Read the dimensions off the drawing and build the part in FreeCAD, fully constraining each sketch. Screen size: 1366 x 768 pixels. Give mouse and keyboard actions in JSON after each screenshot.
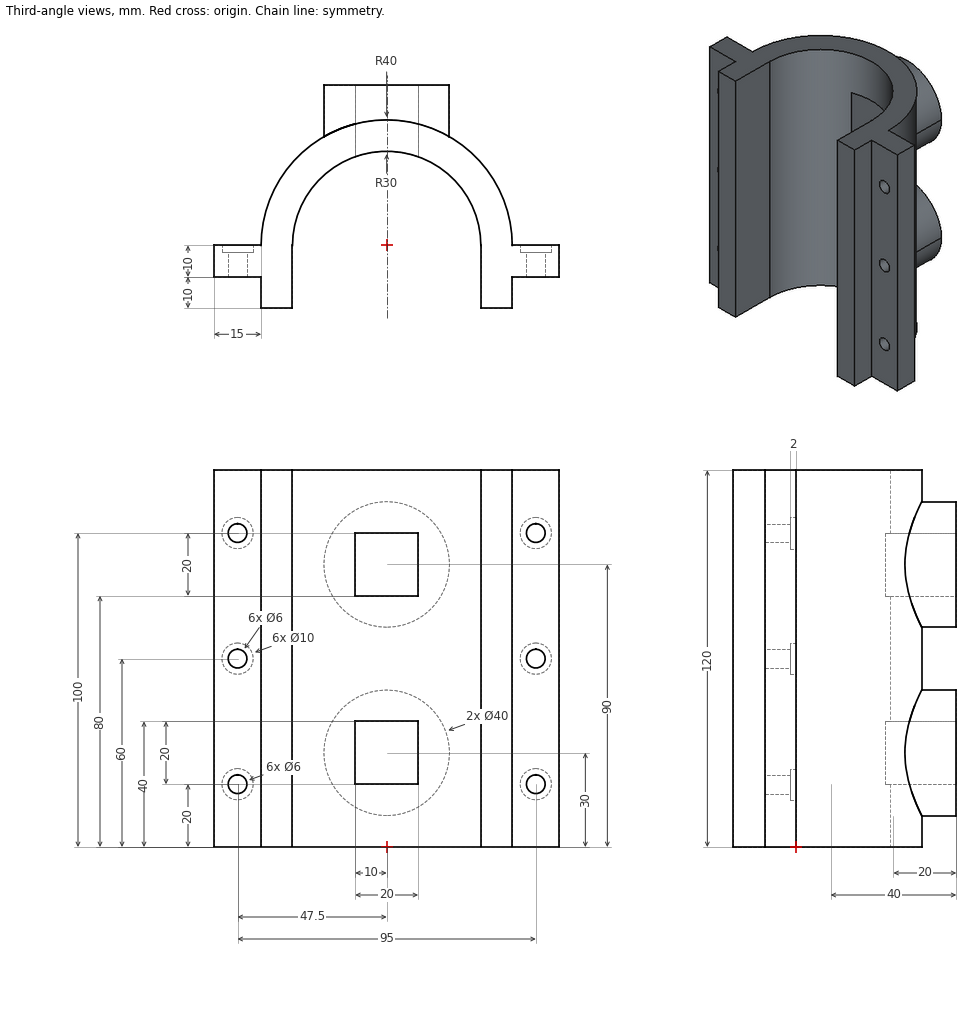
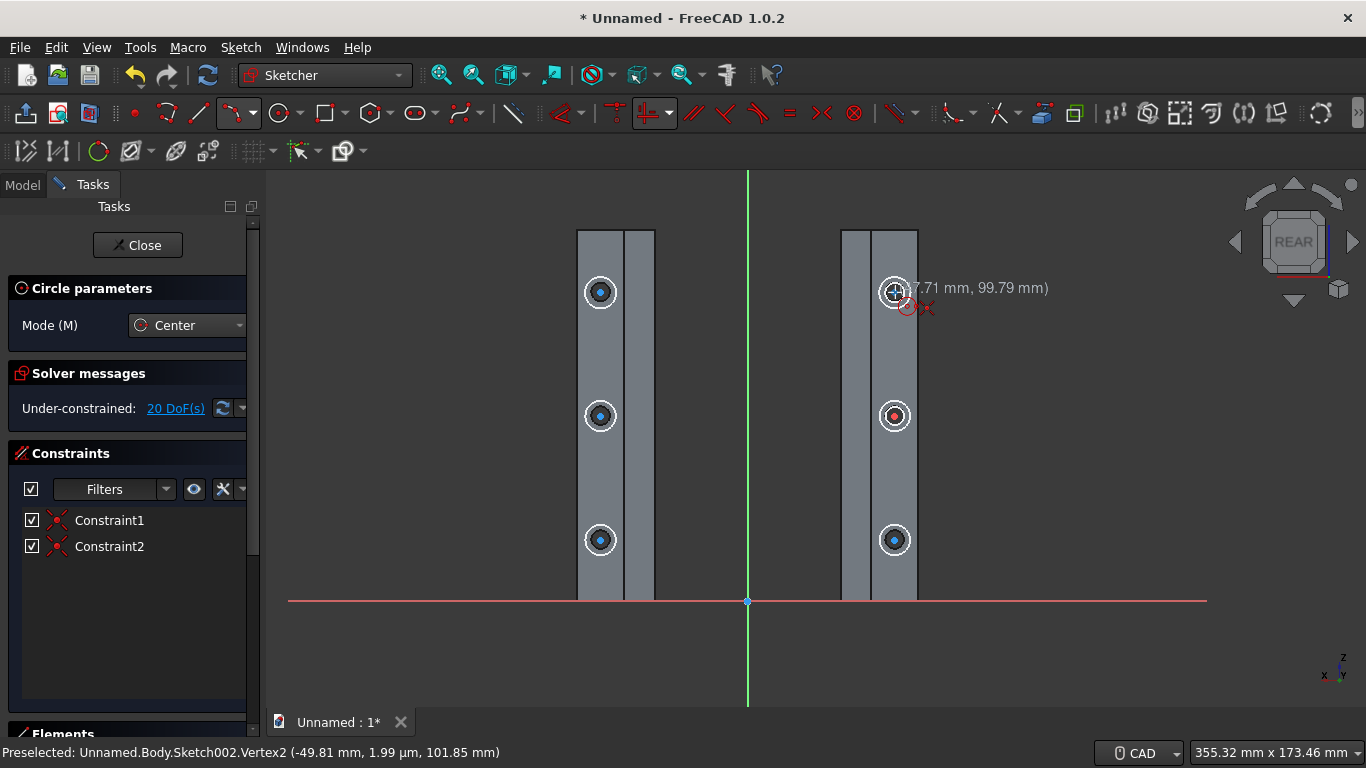
{"action": "scroll", "coordinate": [895, 540], "scroll_direction": "up", "scroll_amount": 5}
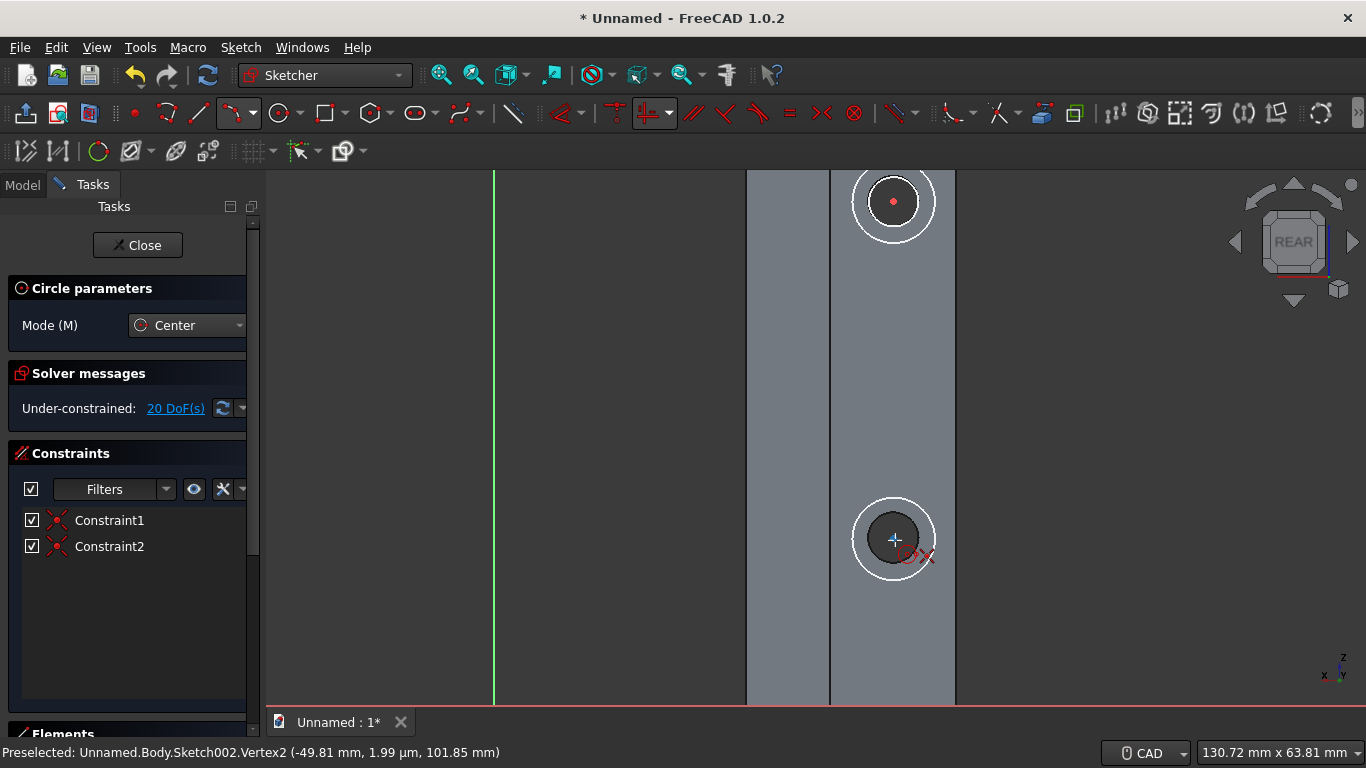
{"action": "left_click", "coordinate": [894, 539]}
{"action": "left_click", "coordinate": [911, 520]}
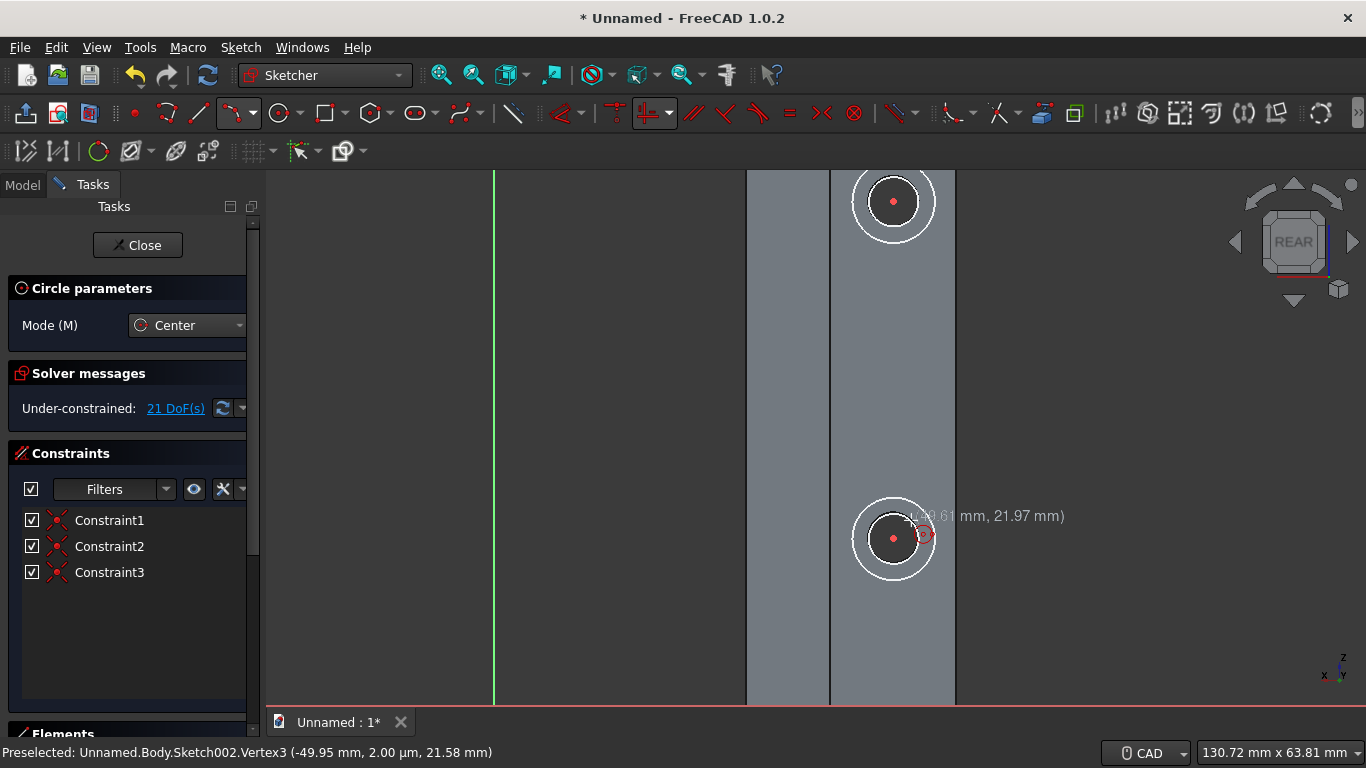
{"action": "scroll", "coordinate": [895, 540], "scroll_direction": "down", "scroll_amount": 5}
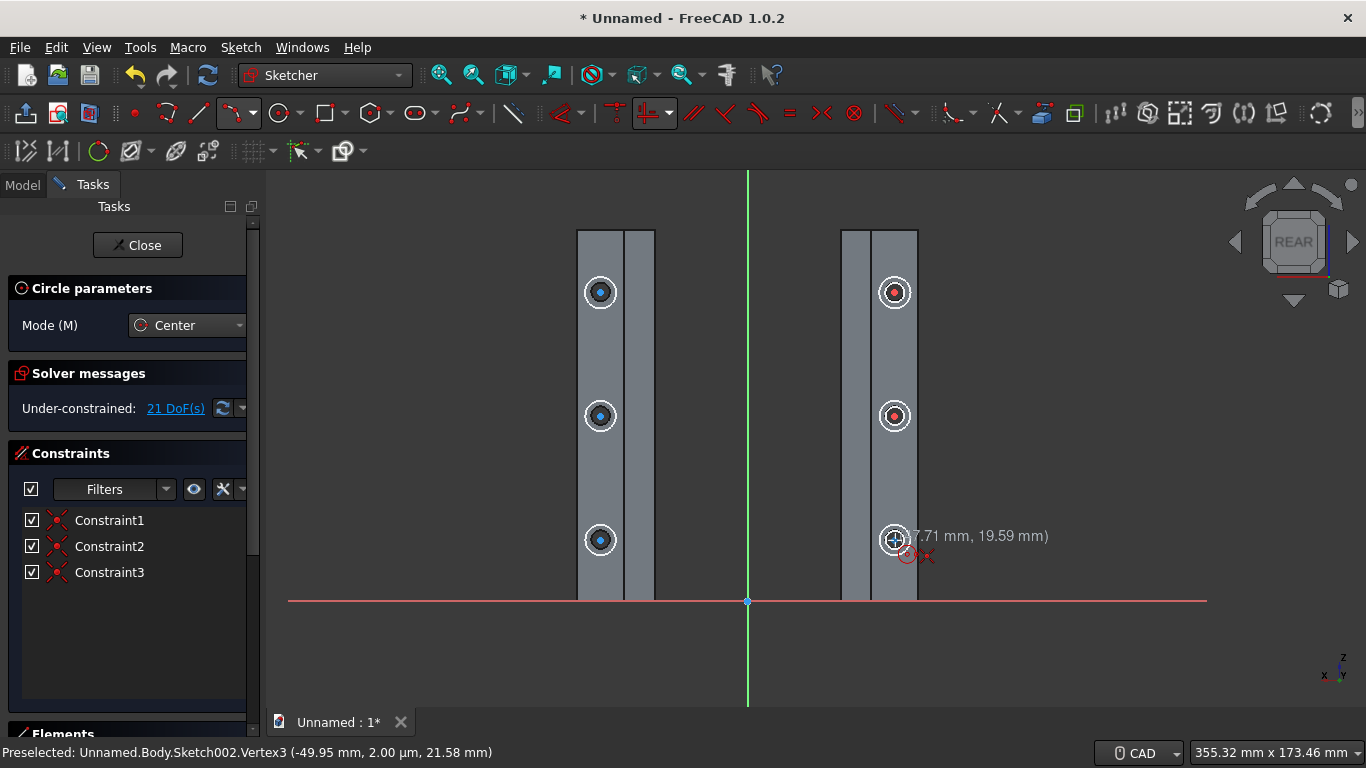
{"action": "scroll", "coordinate": [601, 540], "scroll_direction": "up", "scroll_amount": 5}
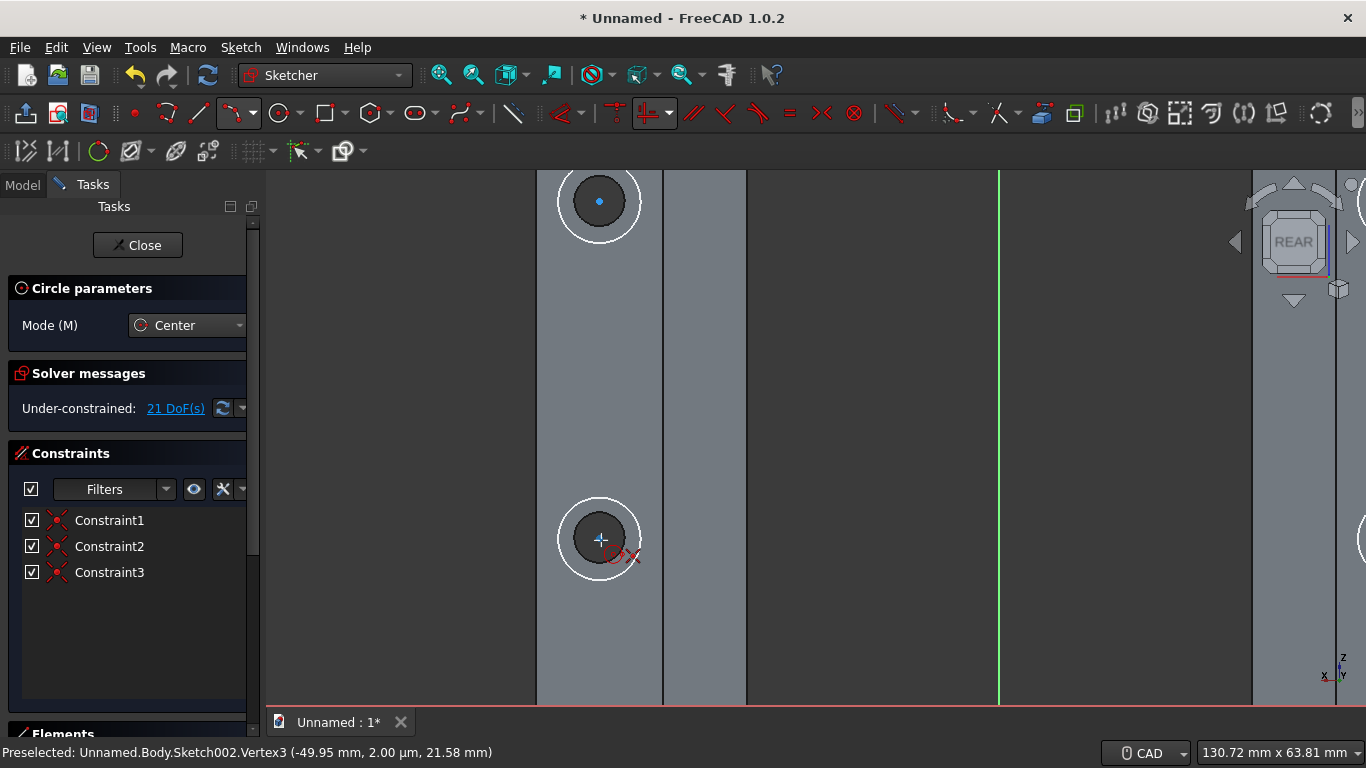
{"action": "left_click", "coordinate": [599, 539]}
{"action": "left_click", "coordinate": [617, 520]}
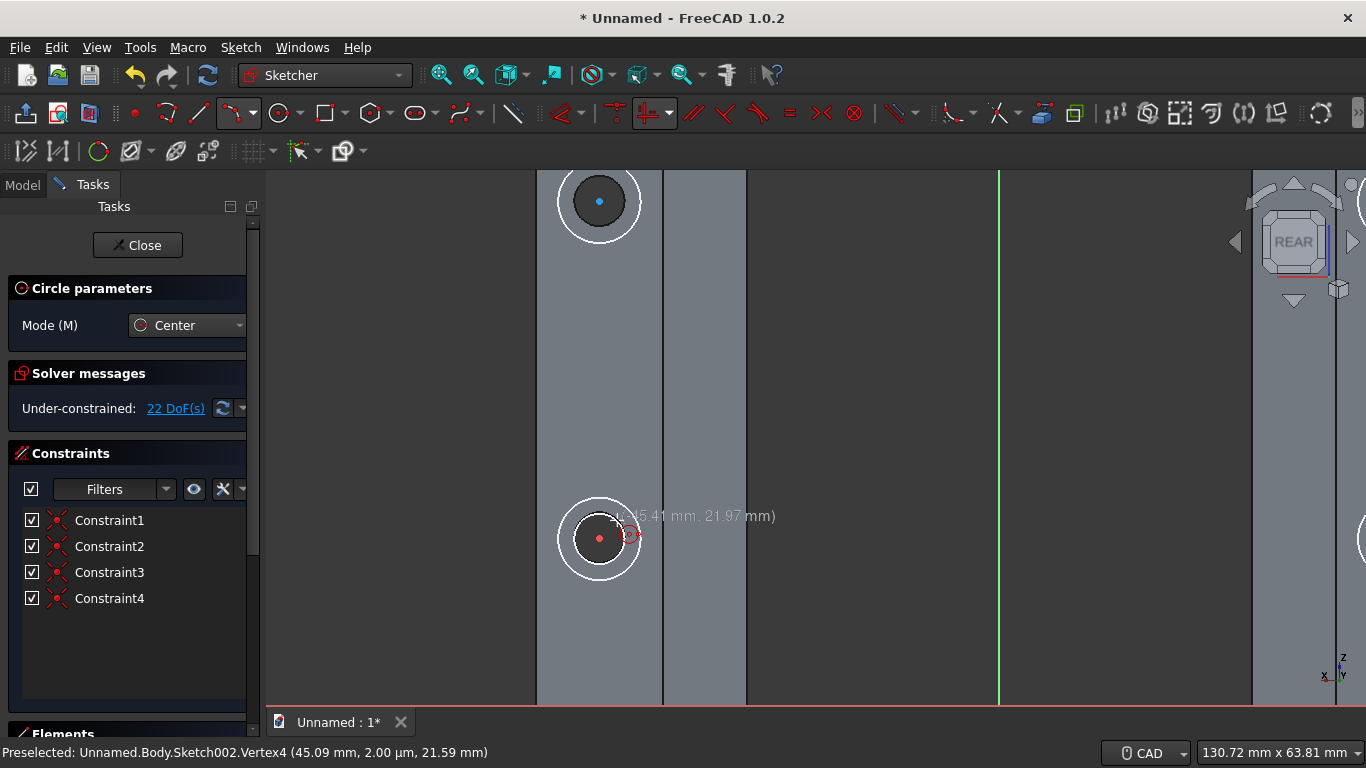
{"action": "left_click", "coordinate": [599, 202]}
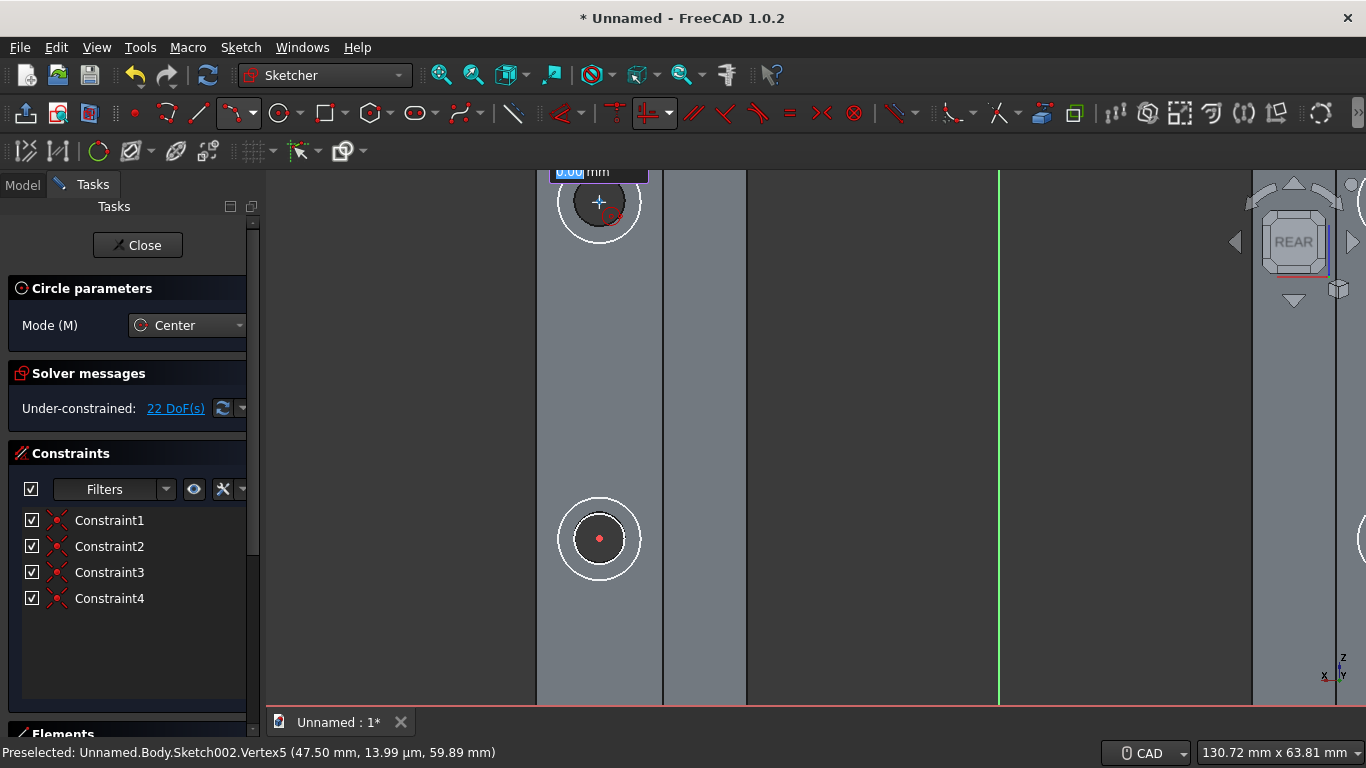
{"action": "scroll", "coordinate": [601, 540], "scroll_direction": "down", "scroll_amount": 5}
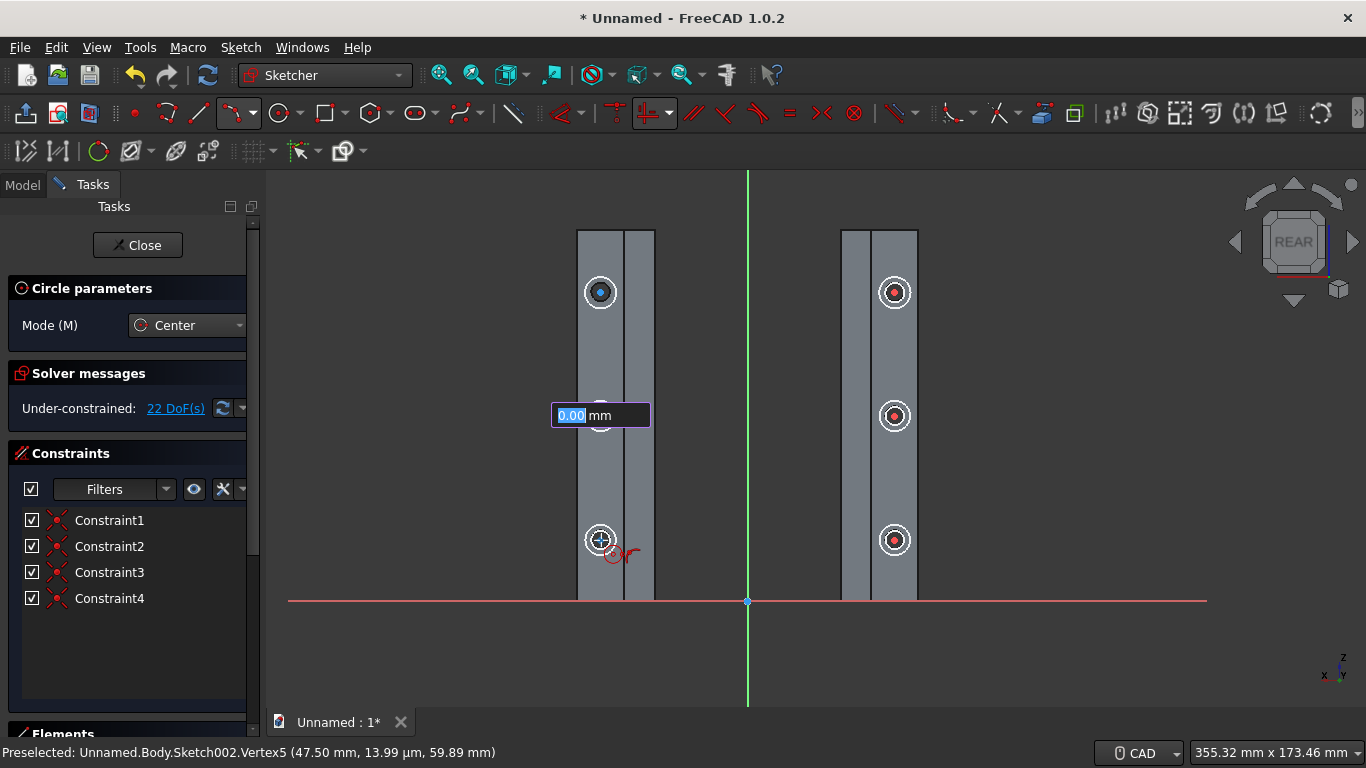
{"action": "scroll", "coordinate": [607, 409], "scroll_direction": "up", "scroll_amount": 5}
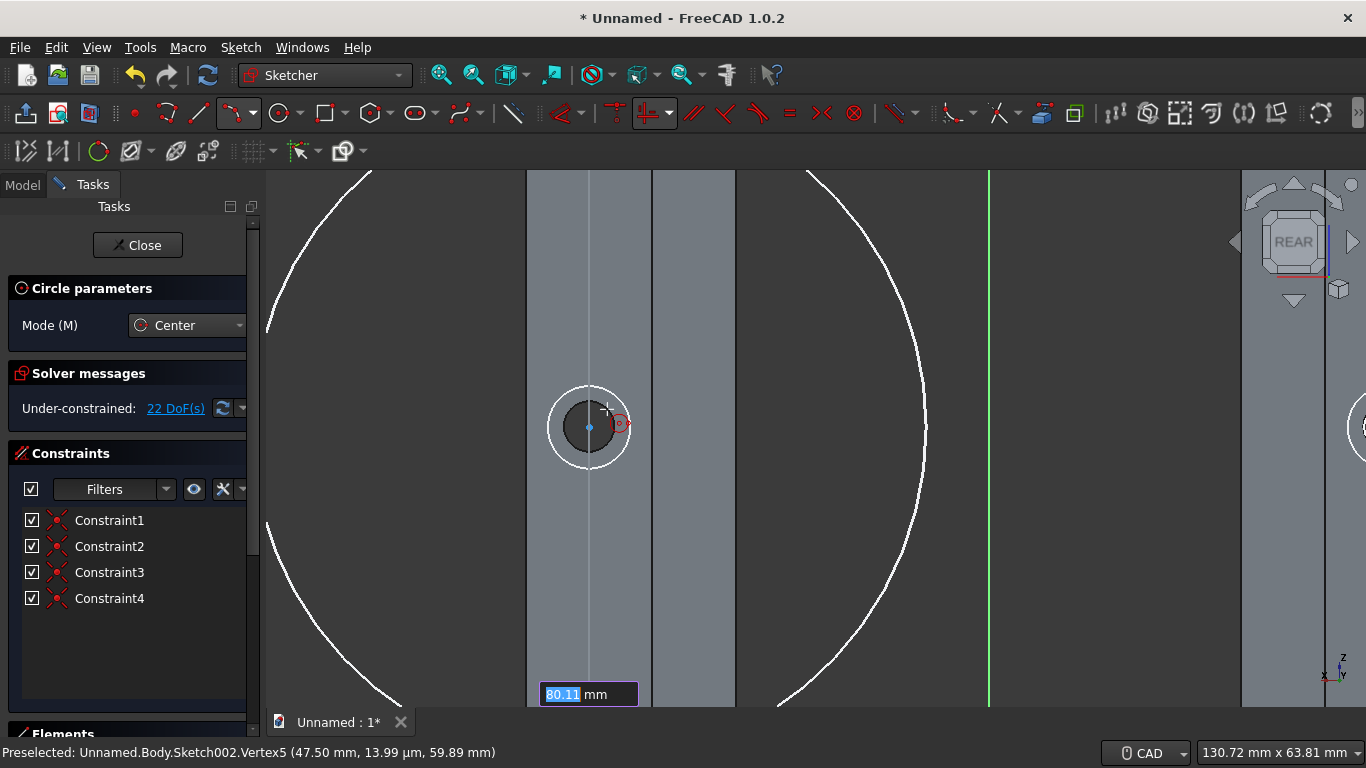
{"action": "left_click", "coordinate": [607, 409]}